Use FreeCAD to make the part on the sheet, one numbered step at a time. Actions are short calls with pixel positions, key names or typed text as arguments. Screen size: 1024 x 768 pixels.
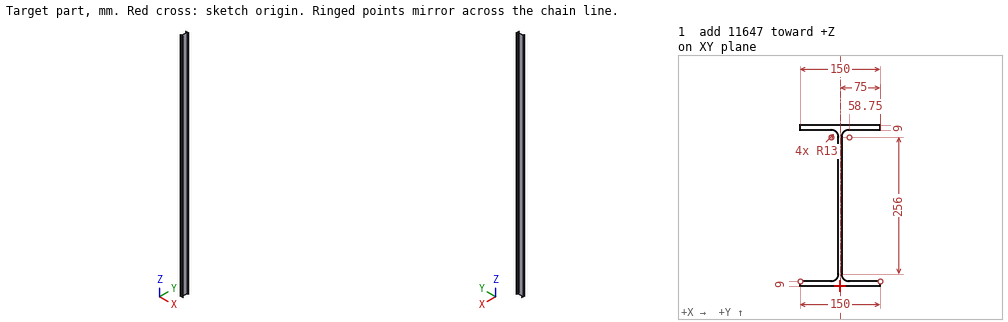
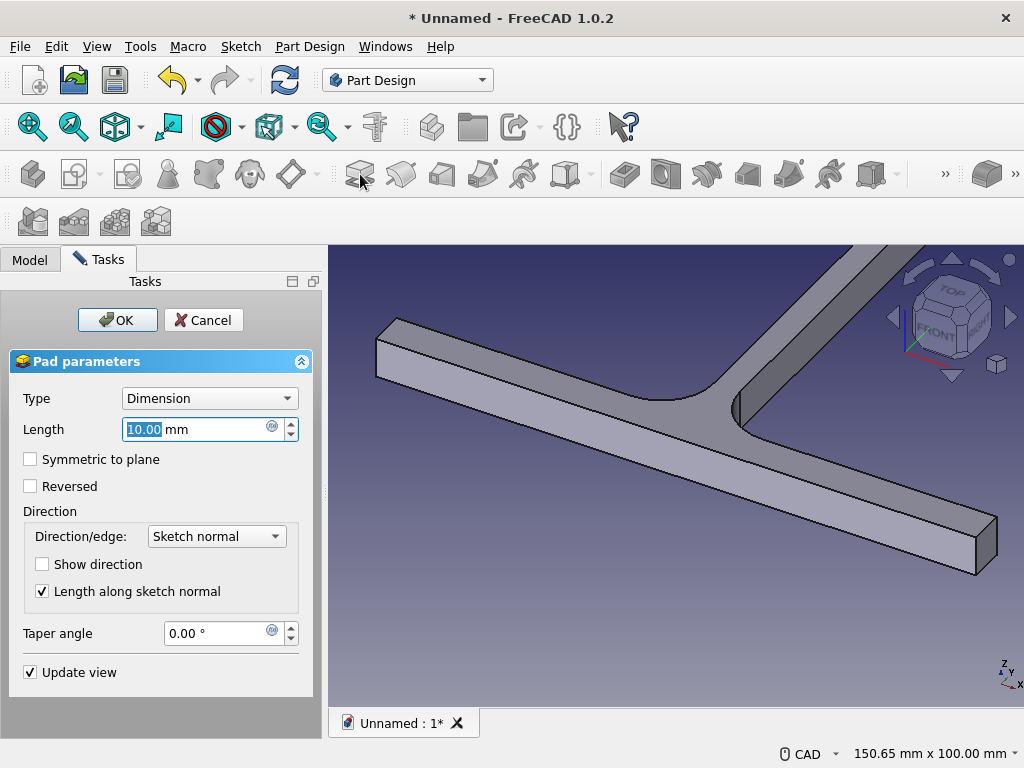
text(11647)
key(Tab)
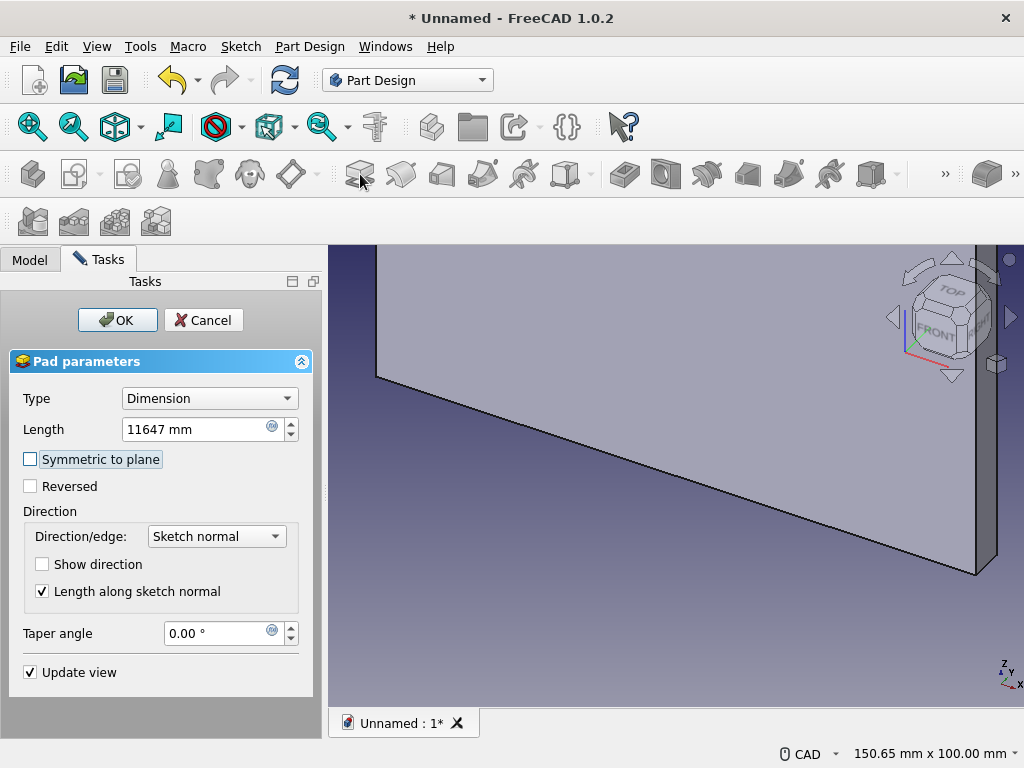
click(118, 320)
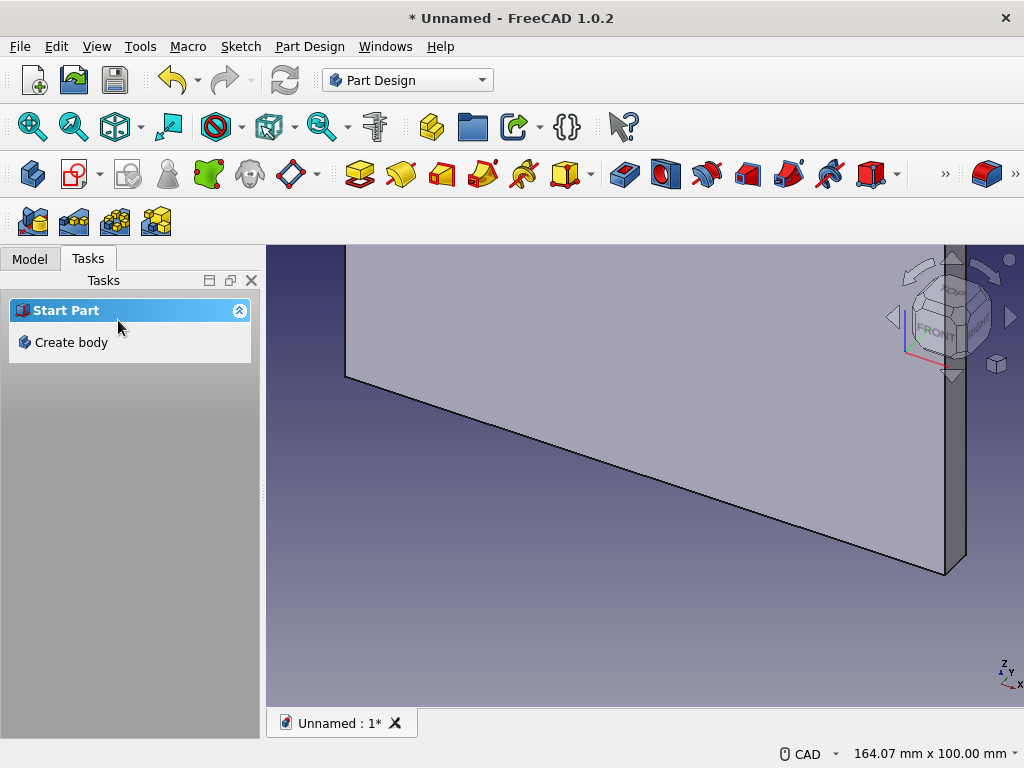
key(0)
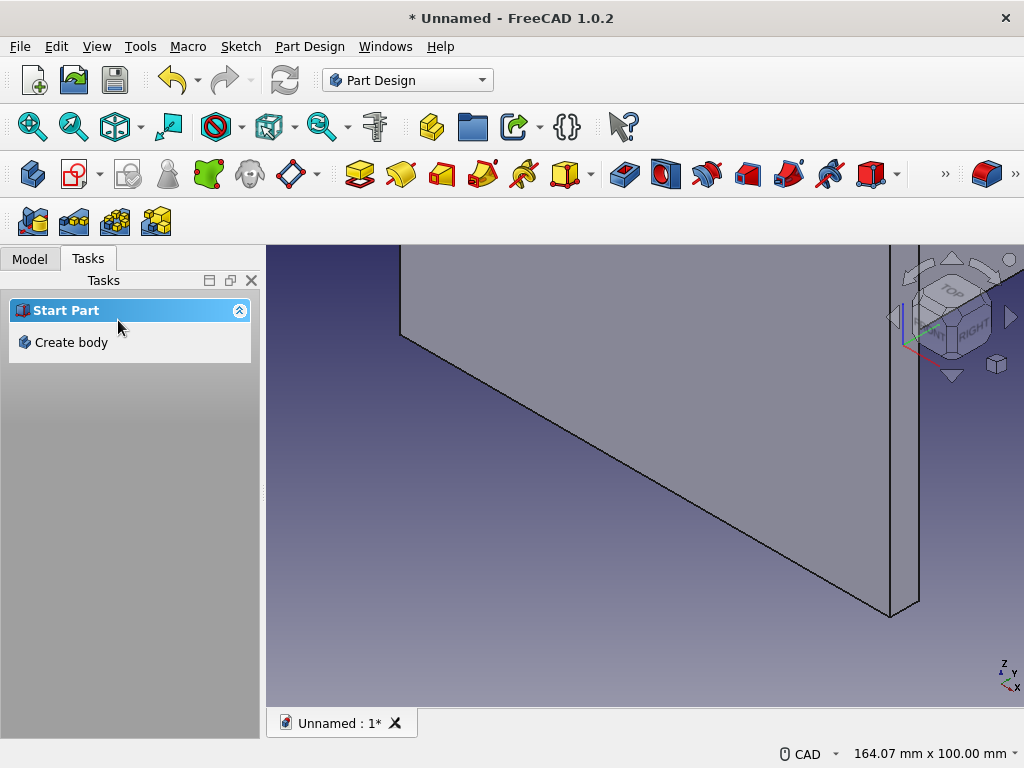
key(v)
key(f)